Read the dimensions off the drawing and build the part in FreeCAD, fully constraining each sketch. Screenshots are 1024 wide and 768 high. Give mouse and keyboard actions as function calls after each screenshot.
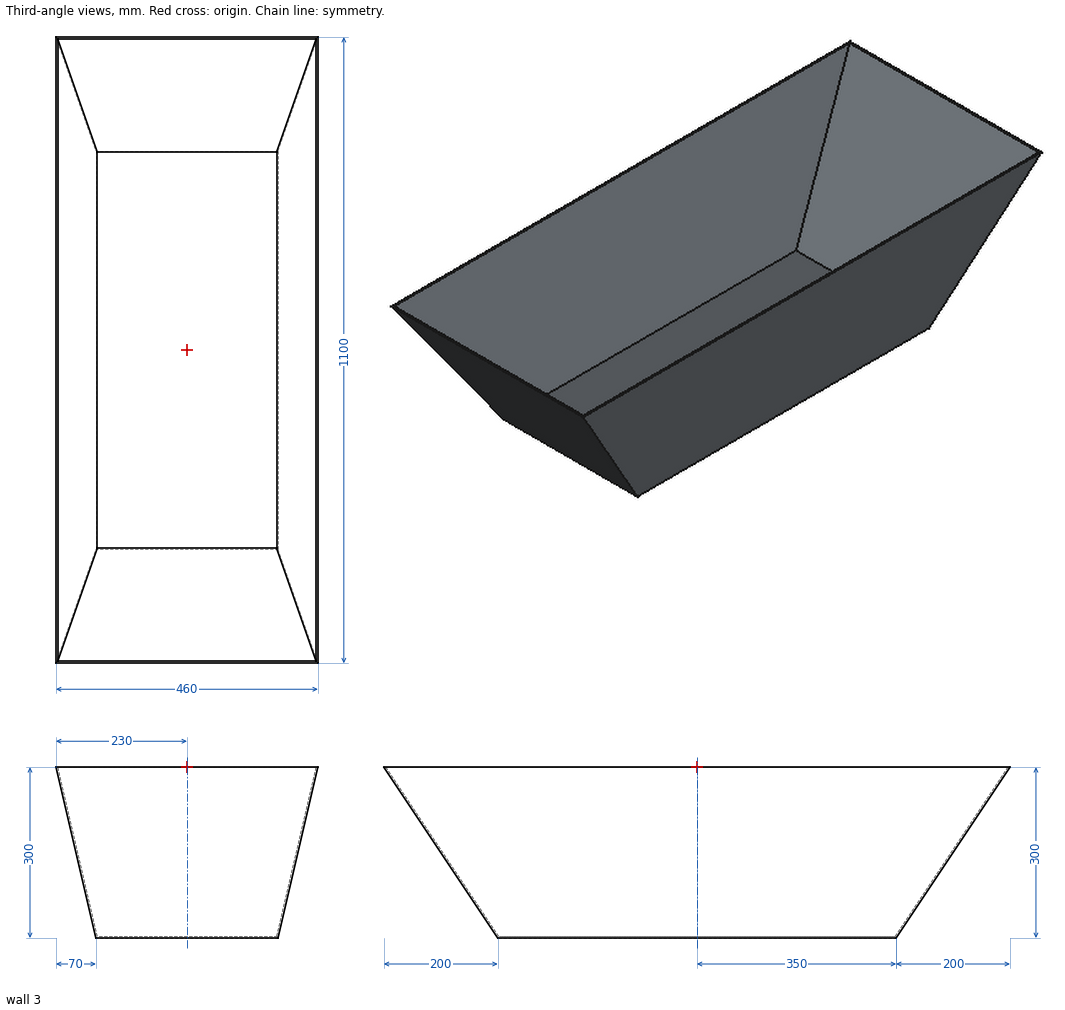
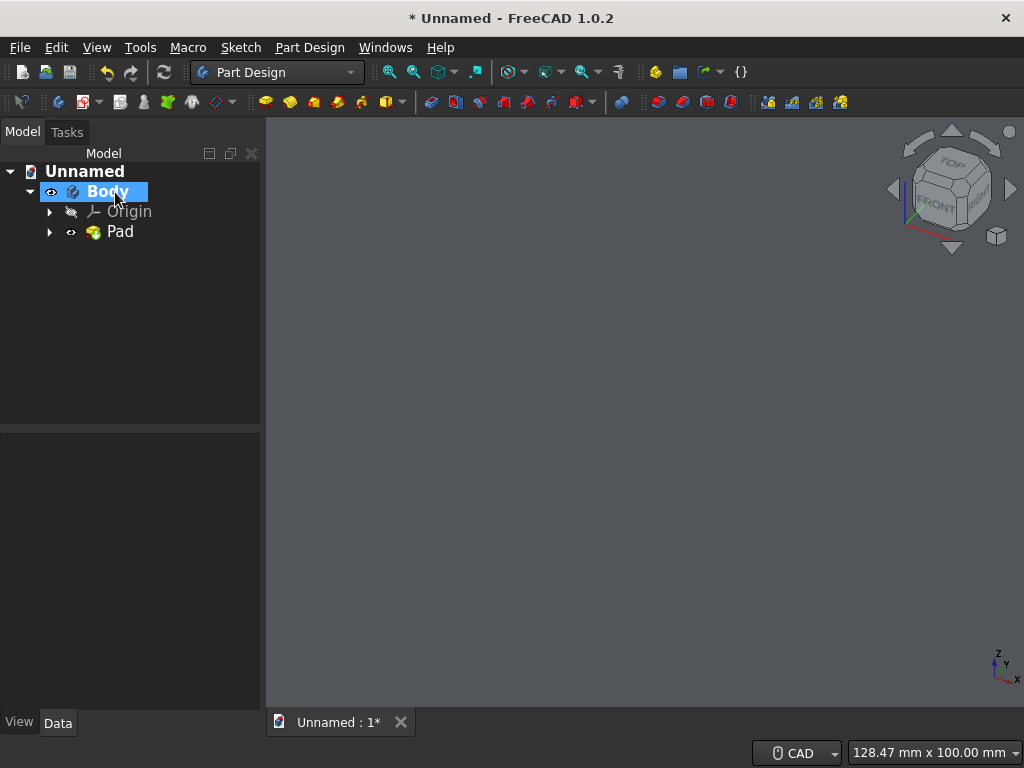
key(v)
key(f)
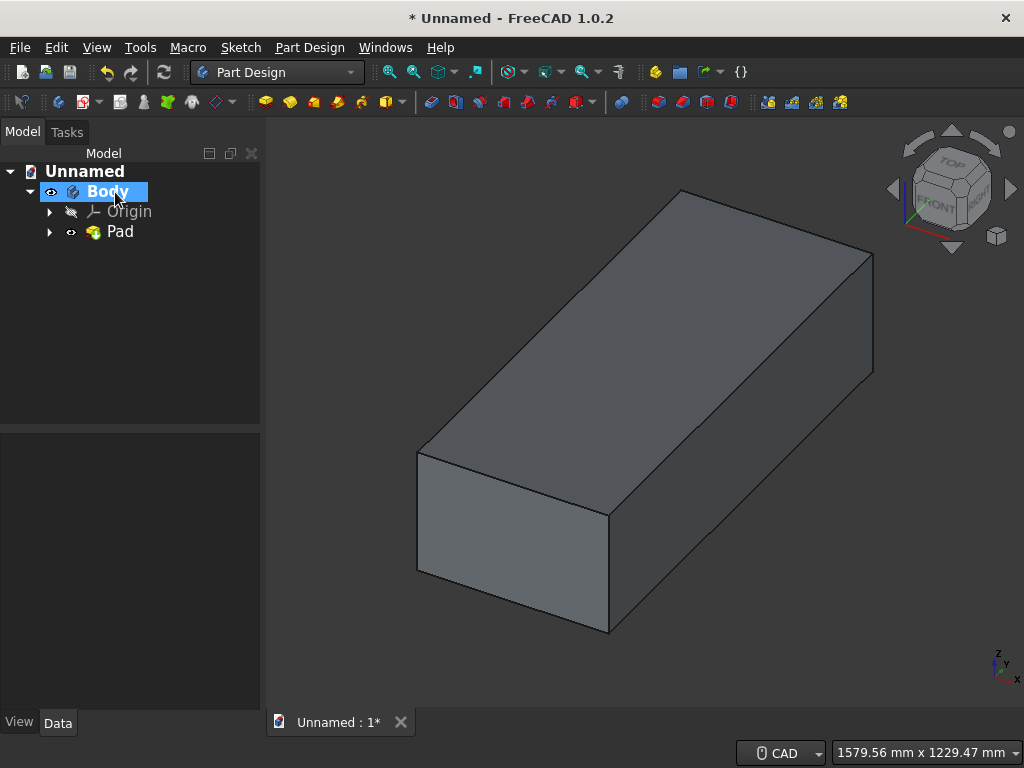
click(816, 368)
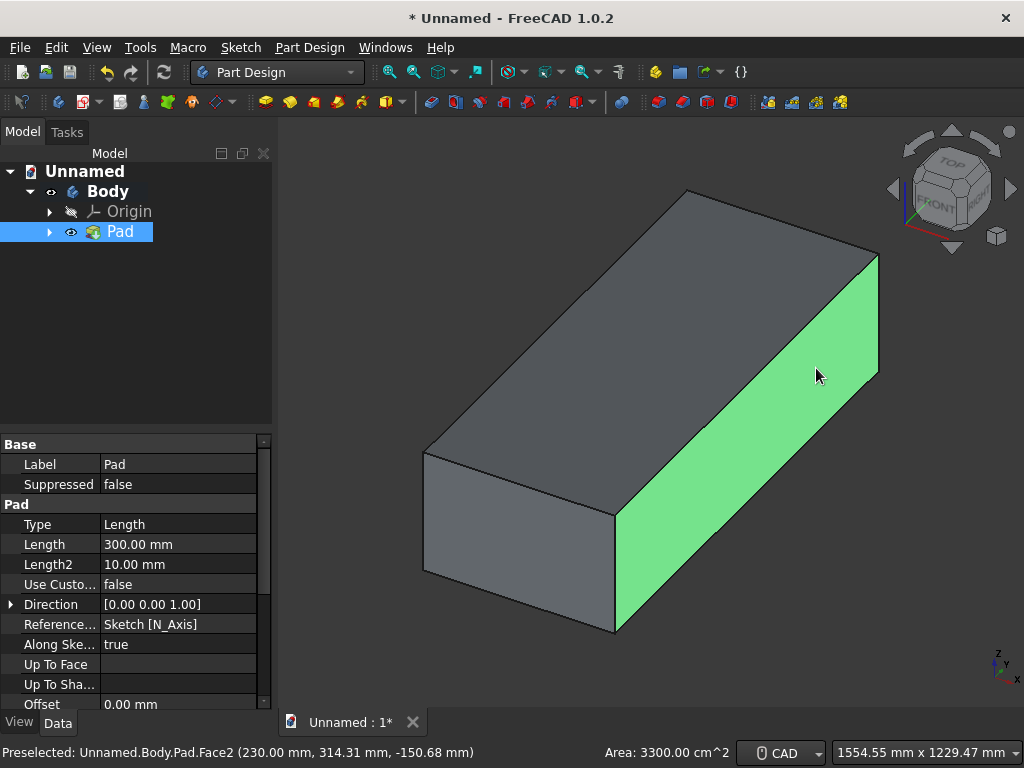
click(84, 102)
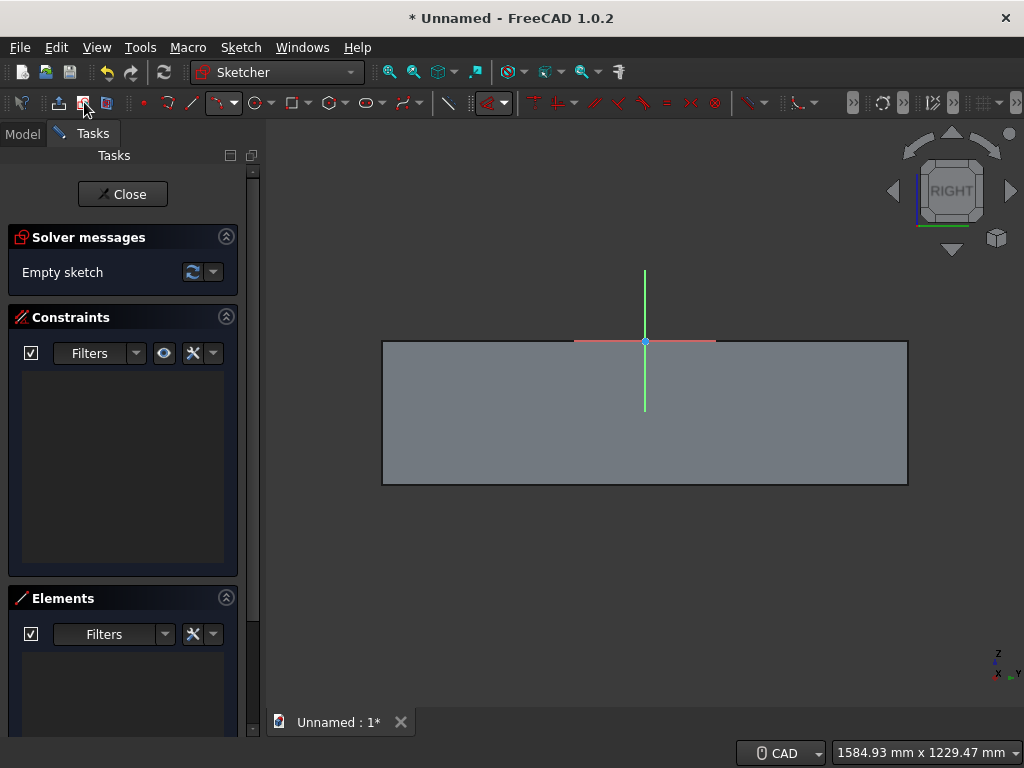
scroll(294, 413, down, 1)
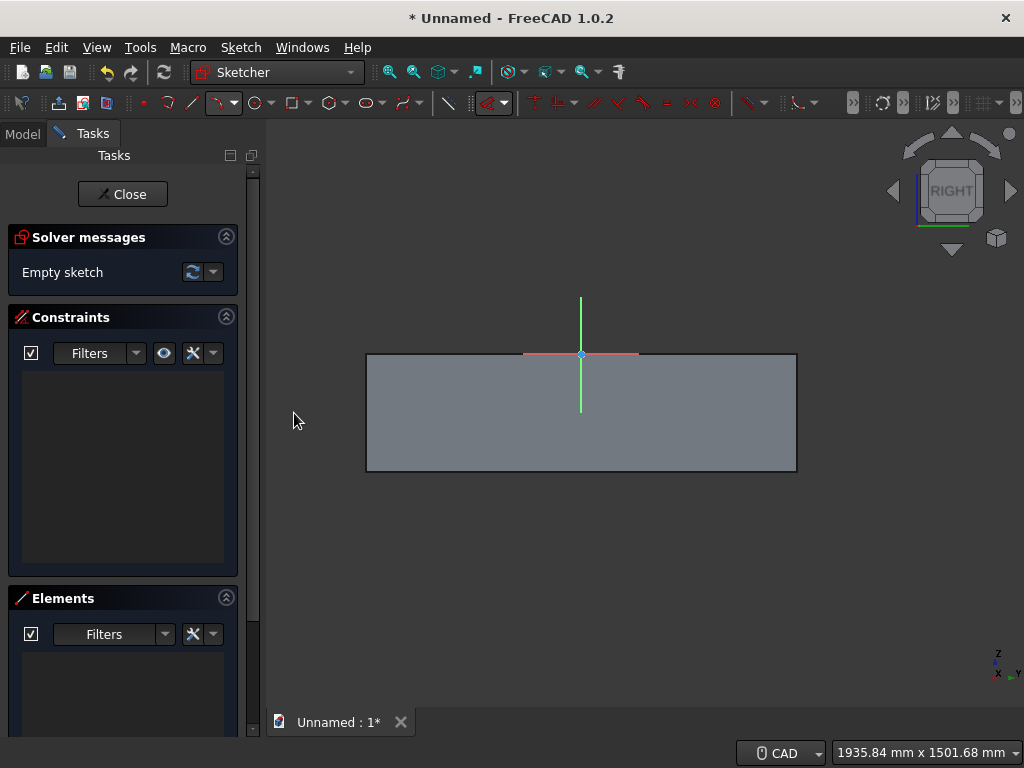
click(168, 104)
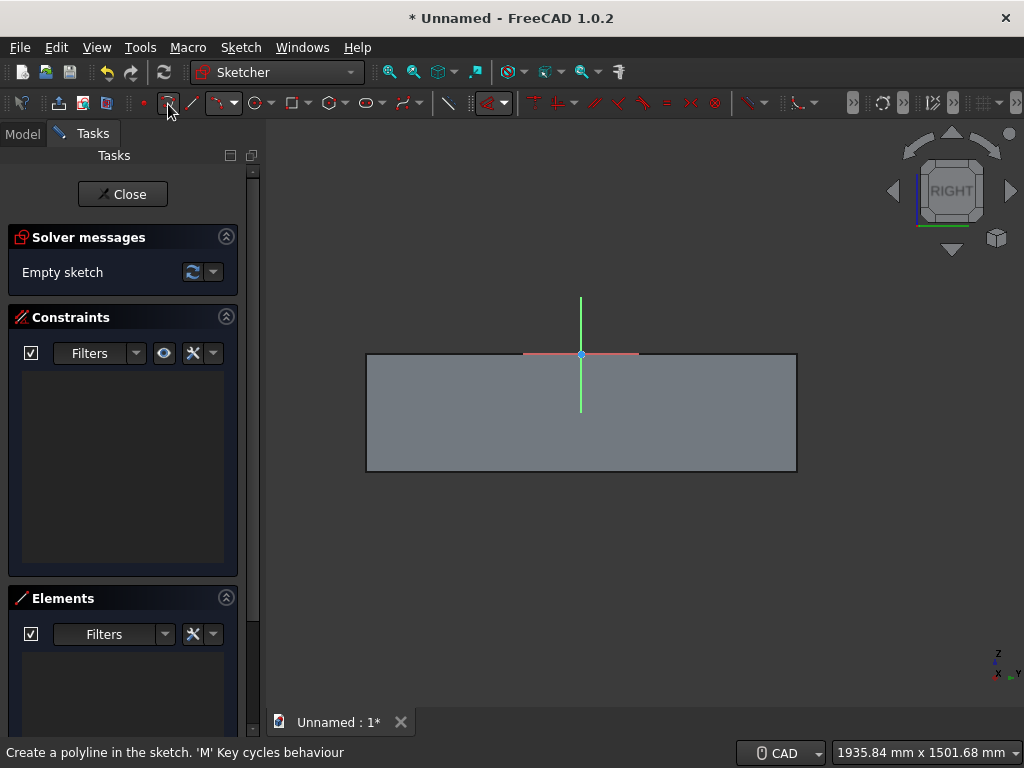
click(718, 472)
click(797, 472)
click(797, 354)
click(718, 473)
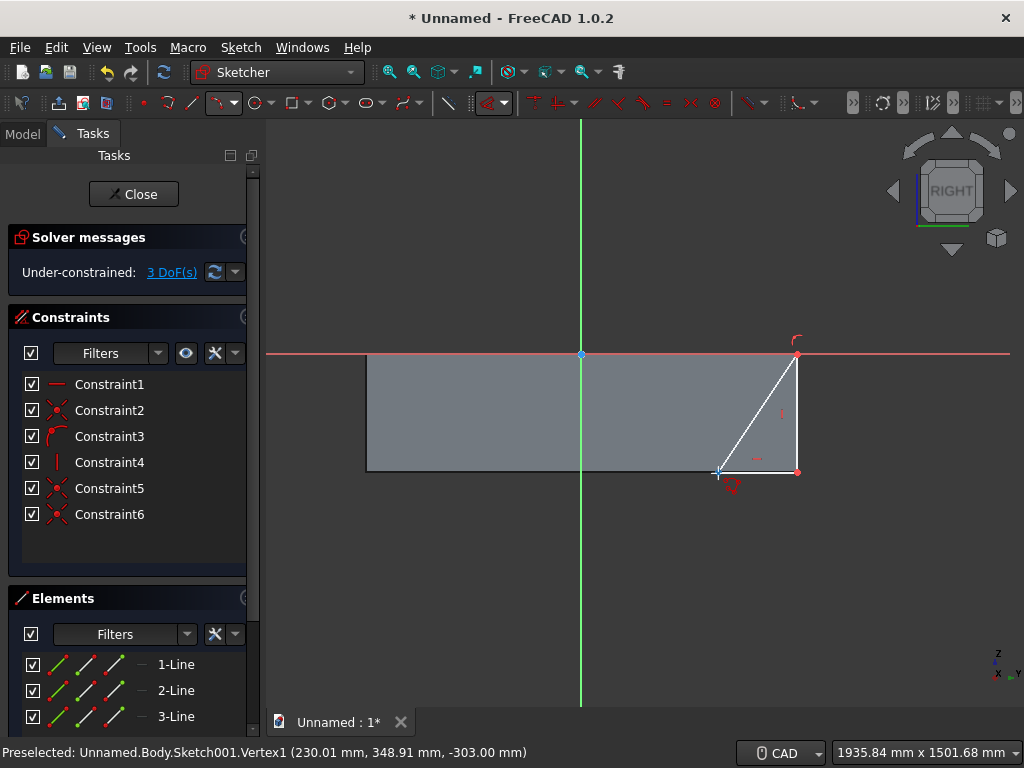
click(444, 472)
click(366, 354)
click(366, 472)
click(444, 473)
key(Escape)
key(Escape)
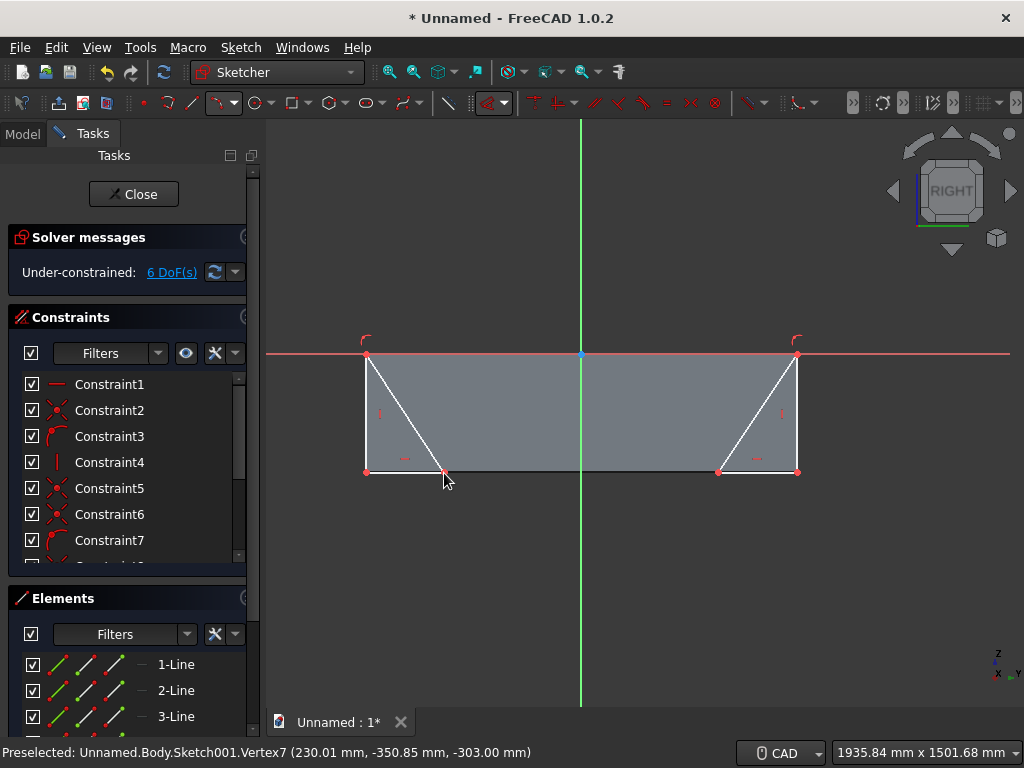
click(718, 473)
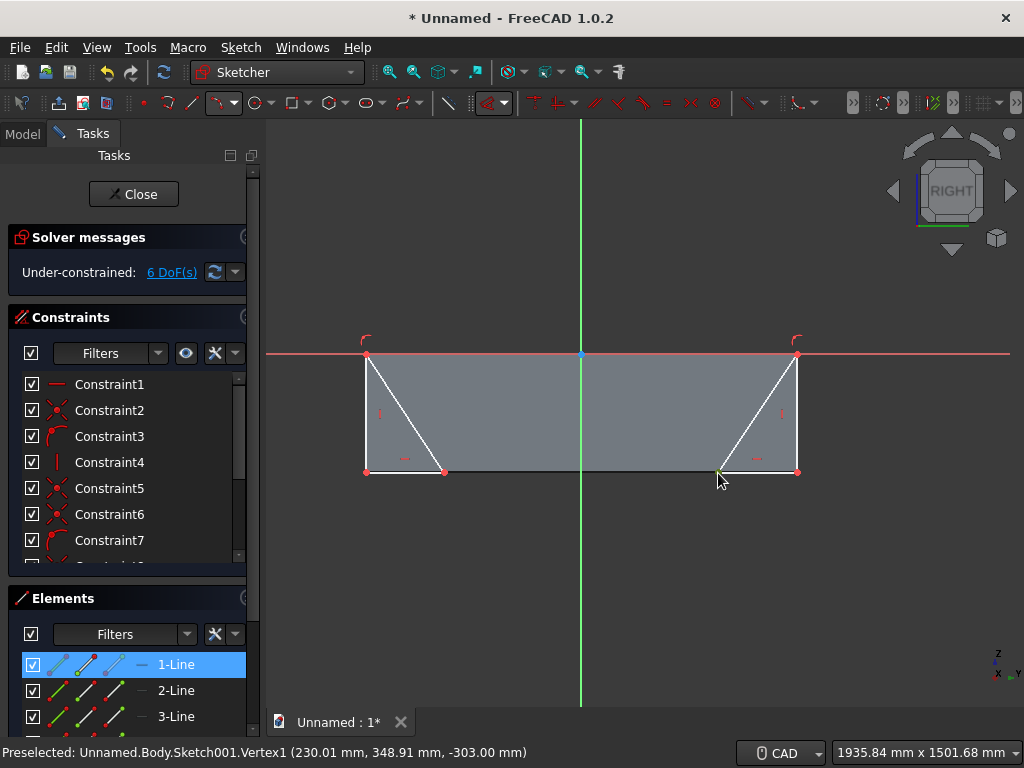
click(444, 473)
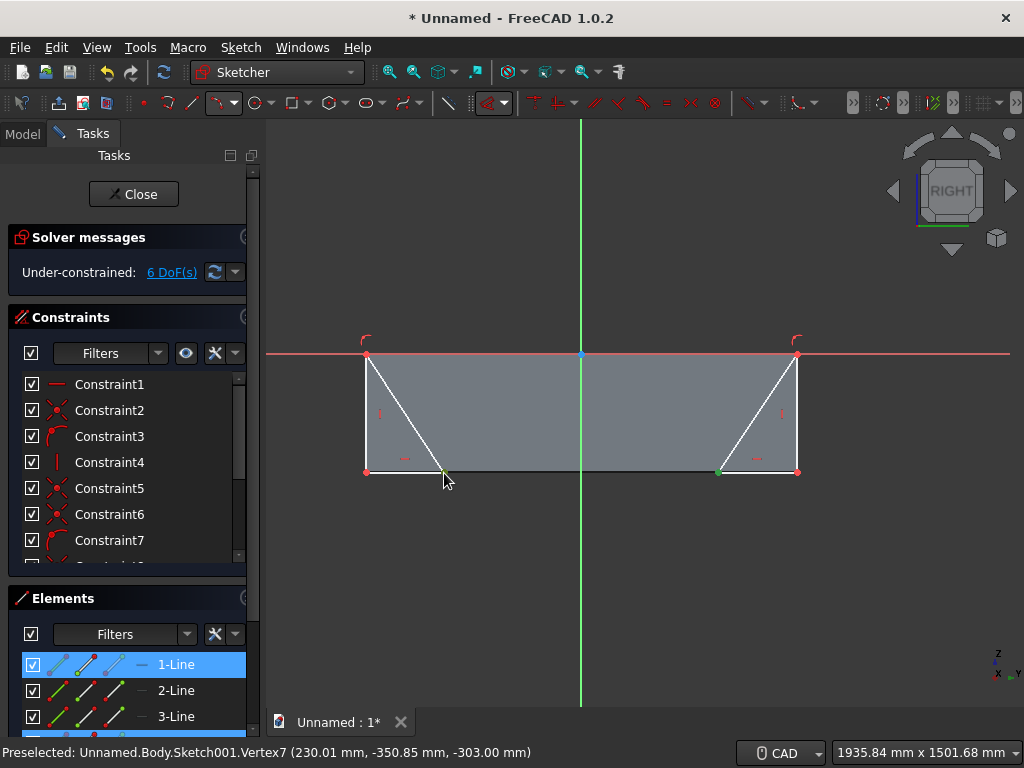
click(581, 641)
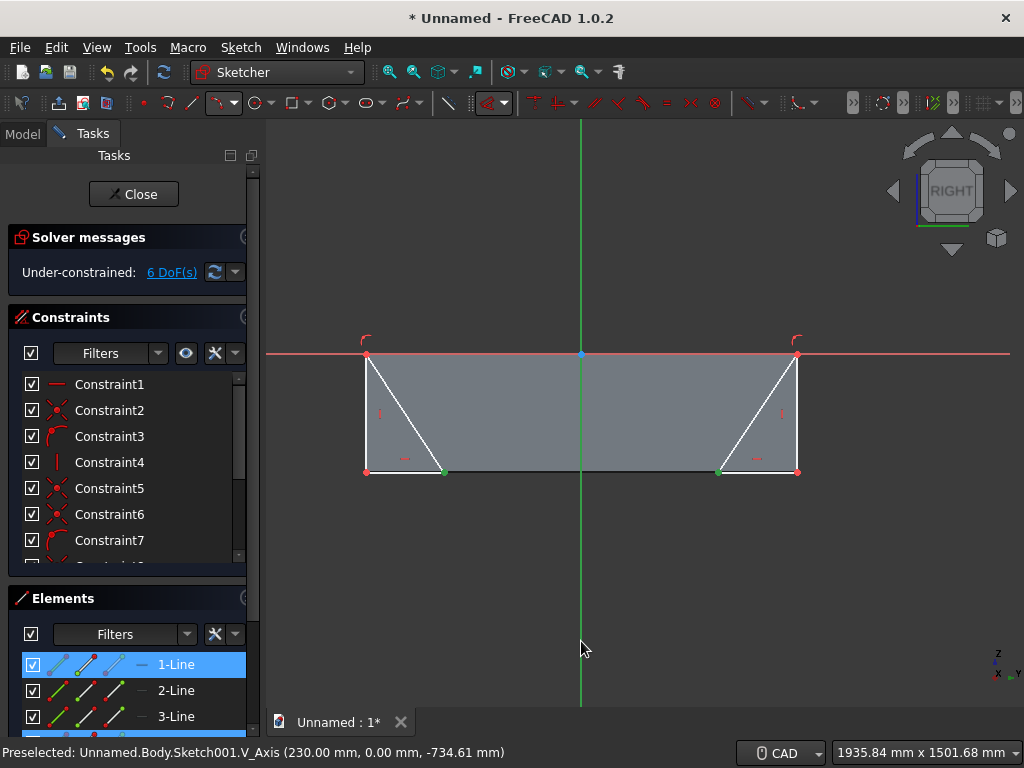
click(692, 104)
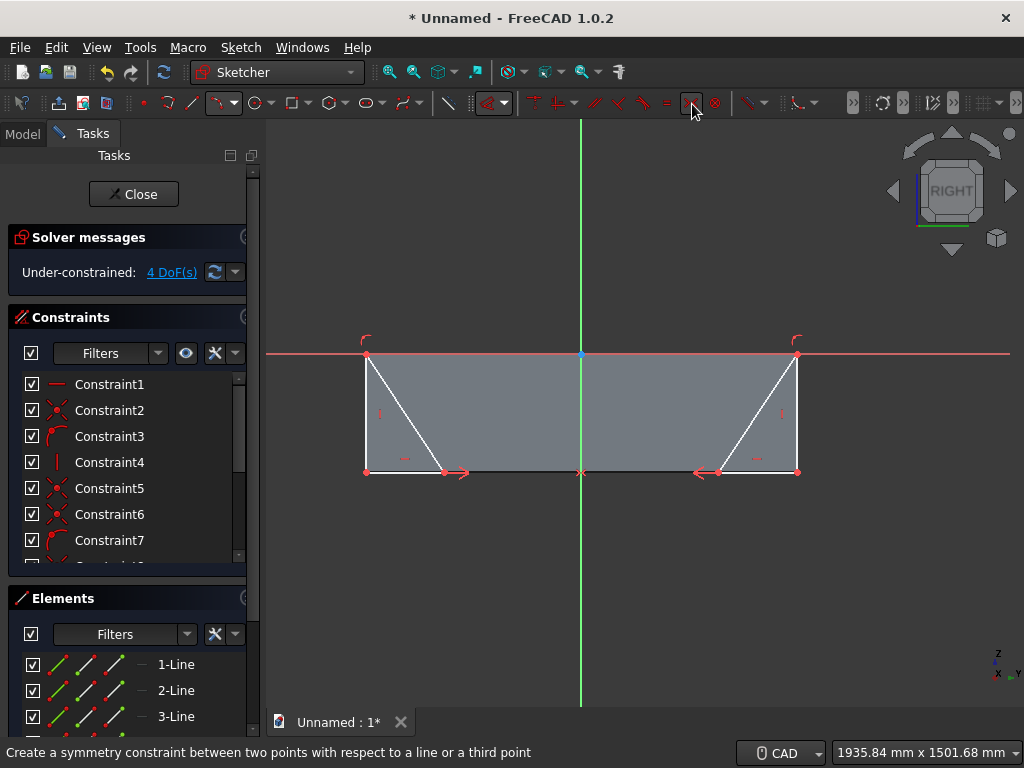
click(488, 104)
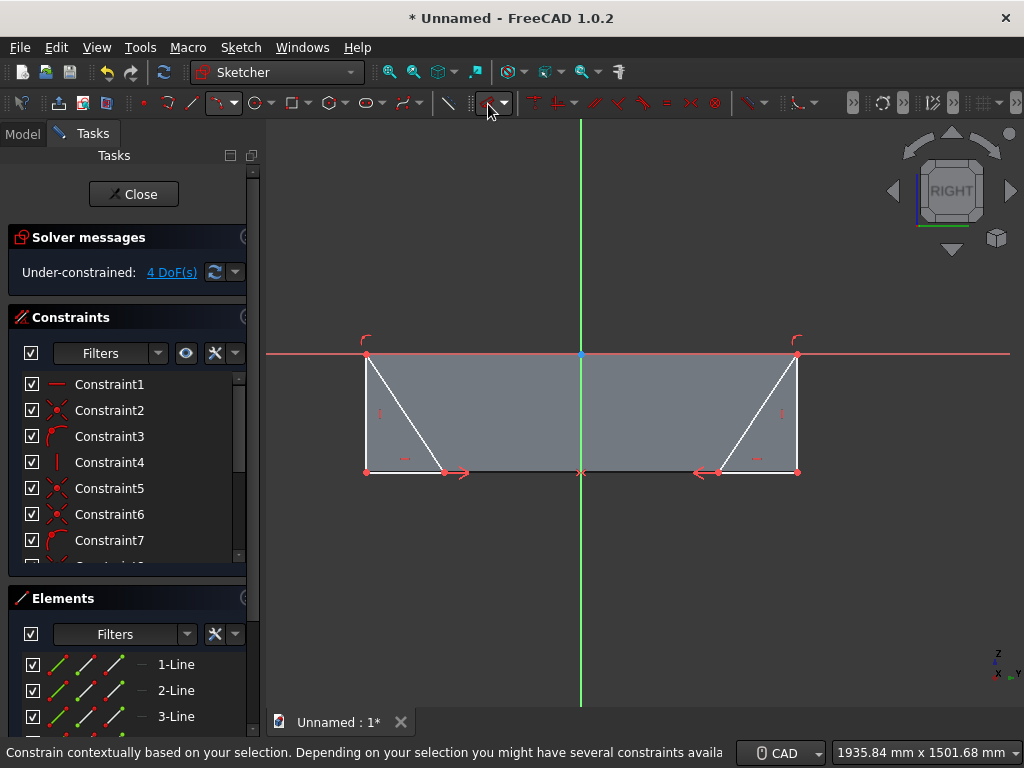
click(742, 473)
click(758, 507)